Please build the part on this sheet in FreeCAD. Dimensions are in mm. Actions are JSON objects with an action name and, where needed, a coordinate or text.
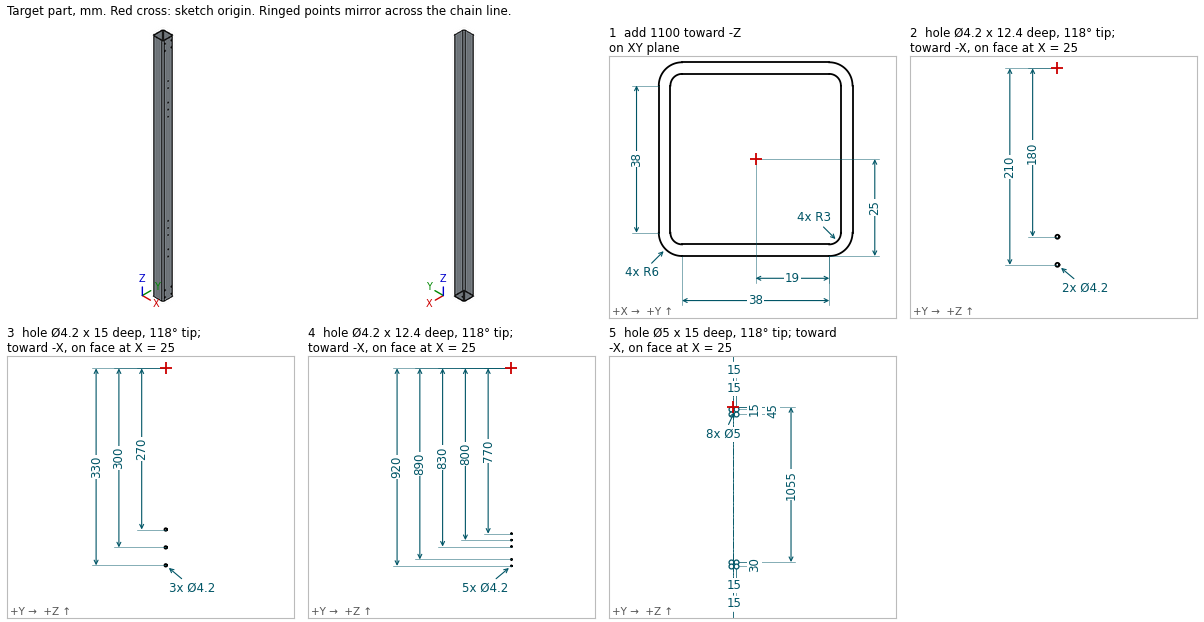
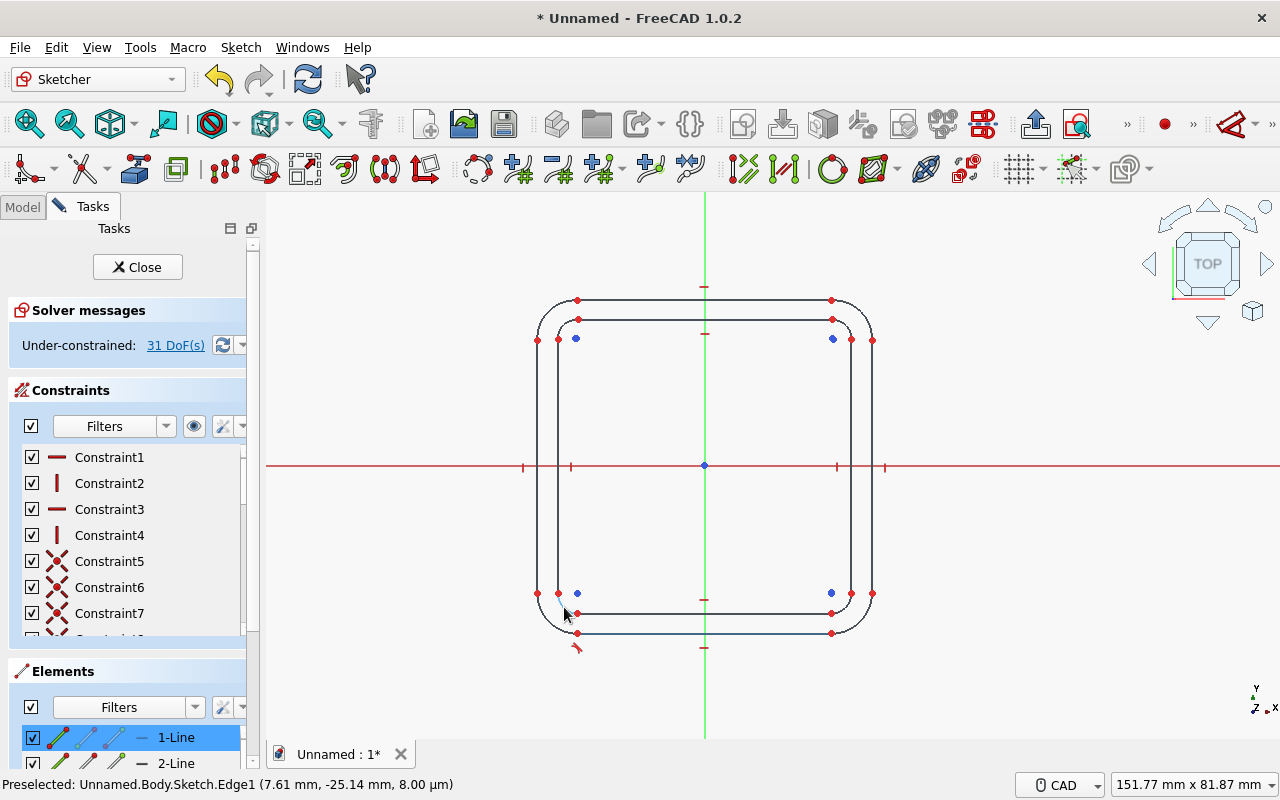
{"action": "left_click", "coordinate": [850, 629]}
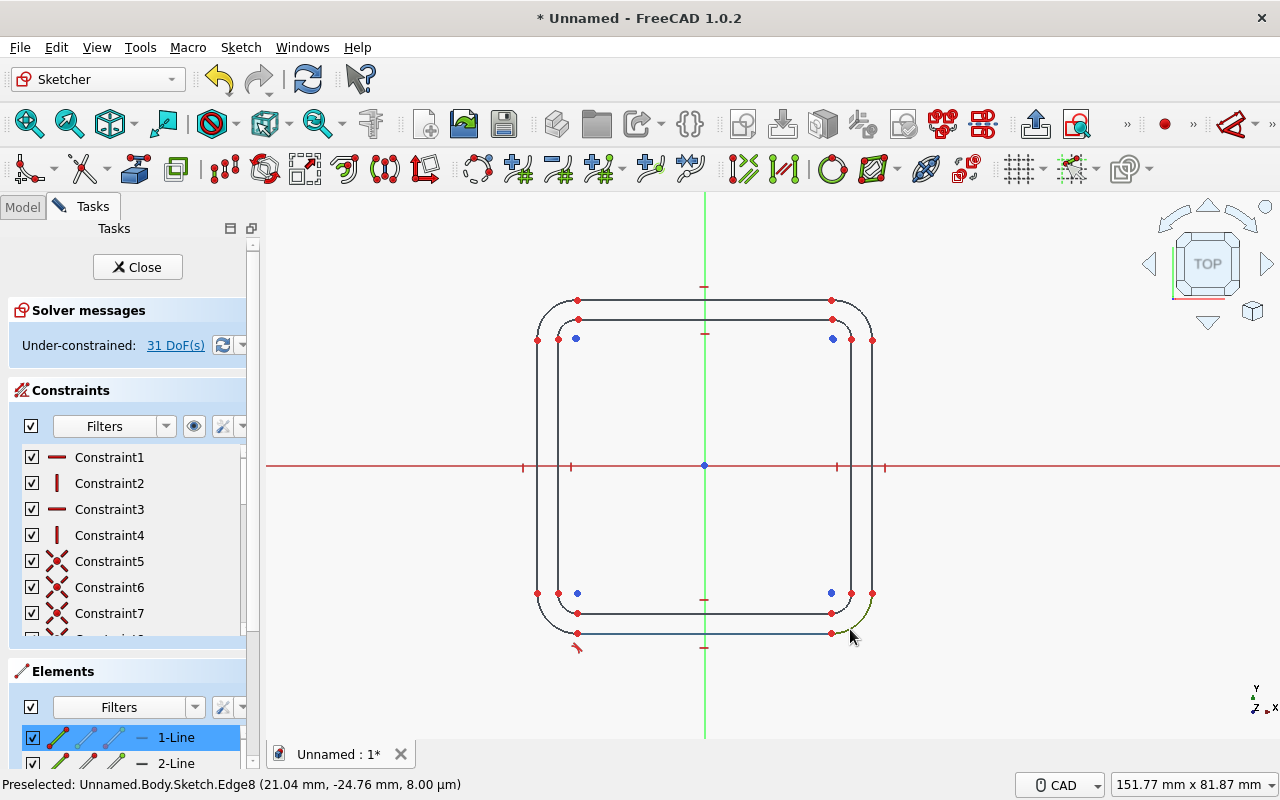
{"action": "key", "text": "t"}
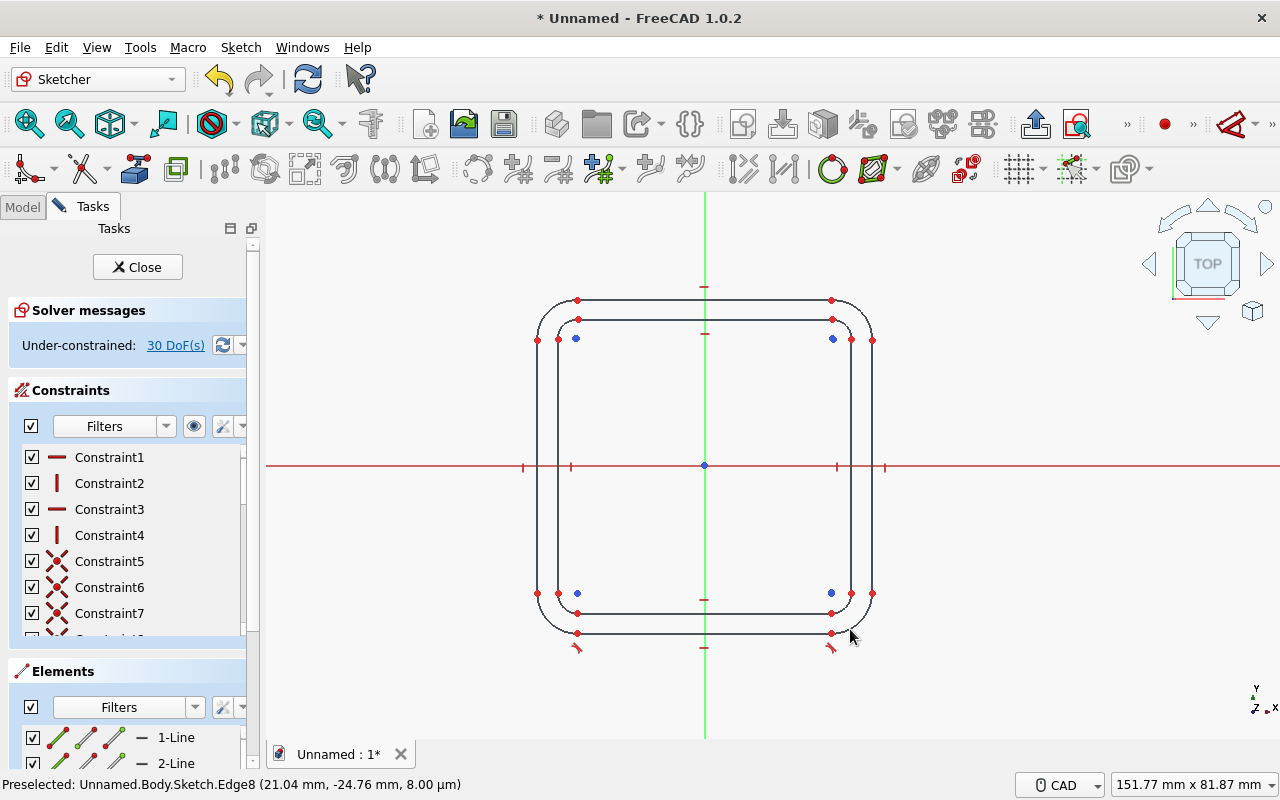
{"action": "left_click", "coordinate": [537, 518]}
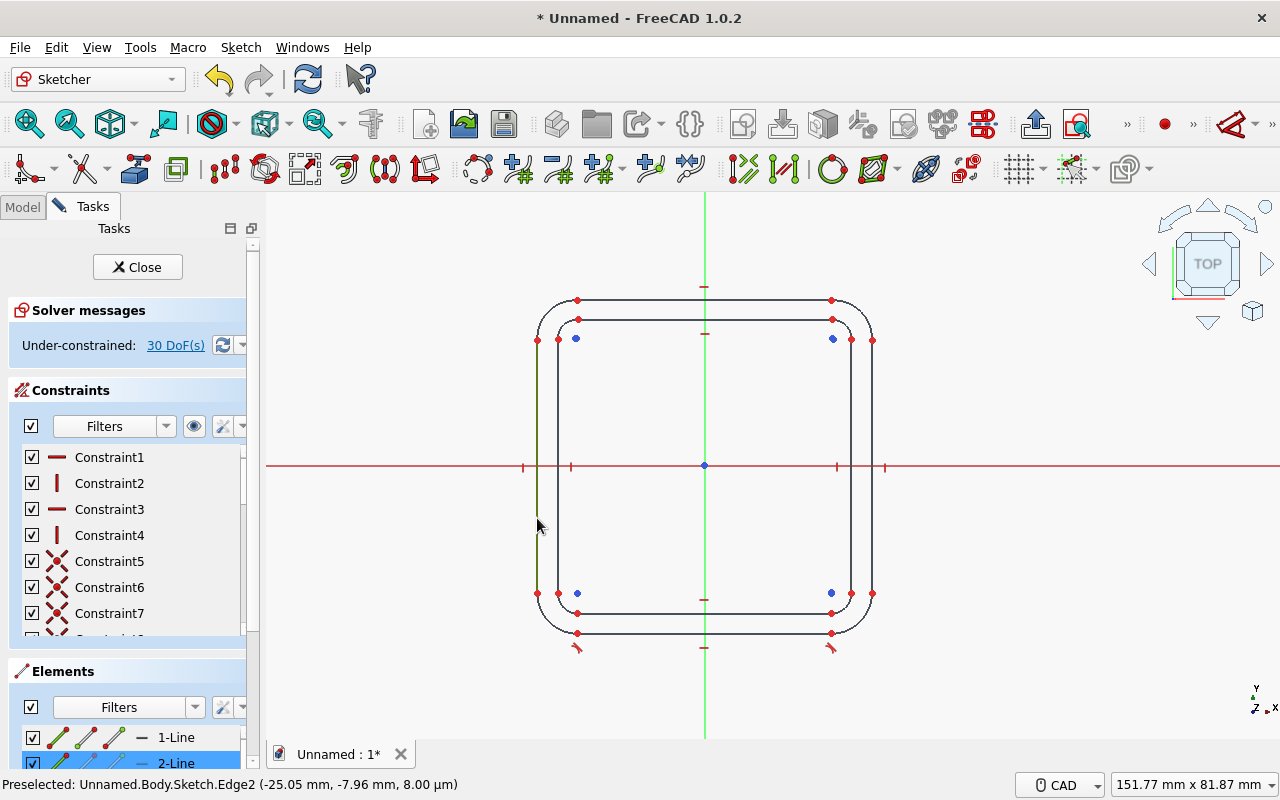
{"action": "left_click", "coordinate": [542, 612]}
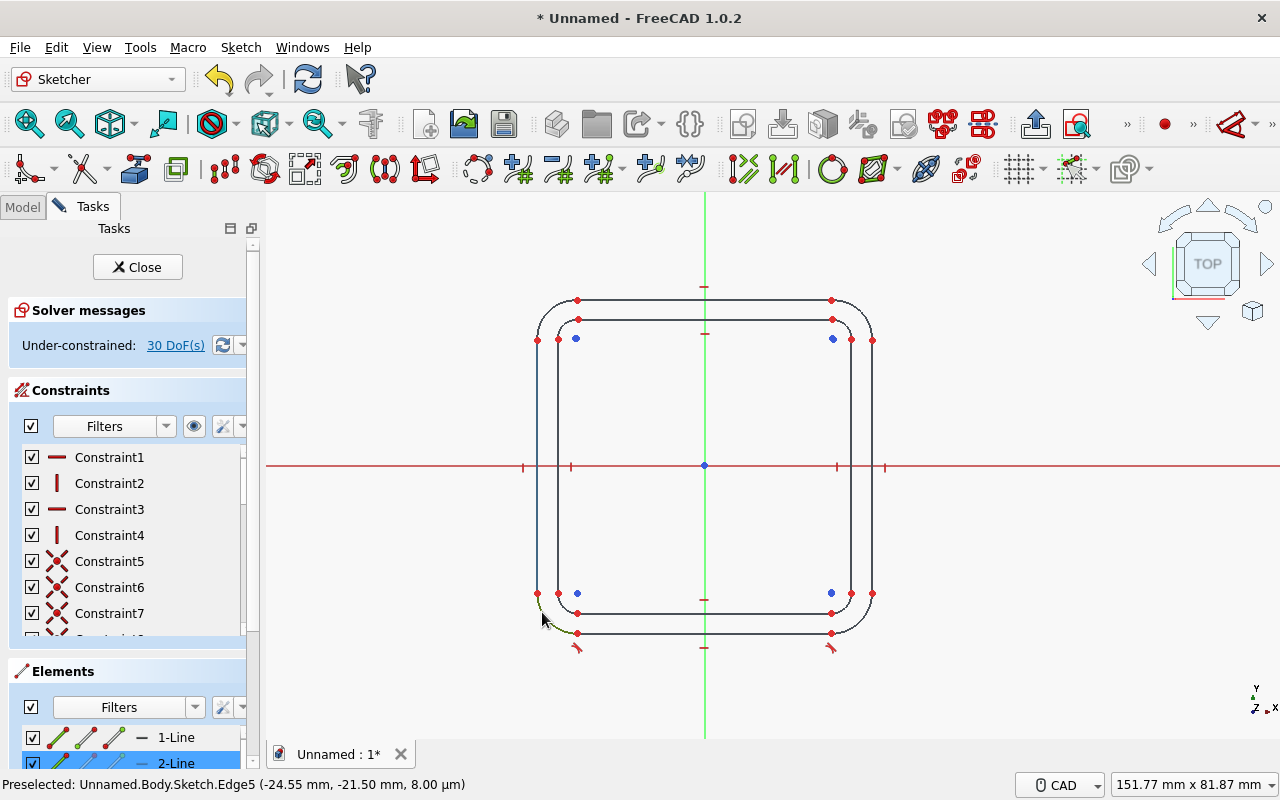
{"action": "key", "text": "t"}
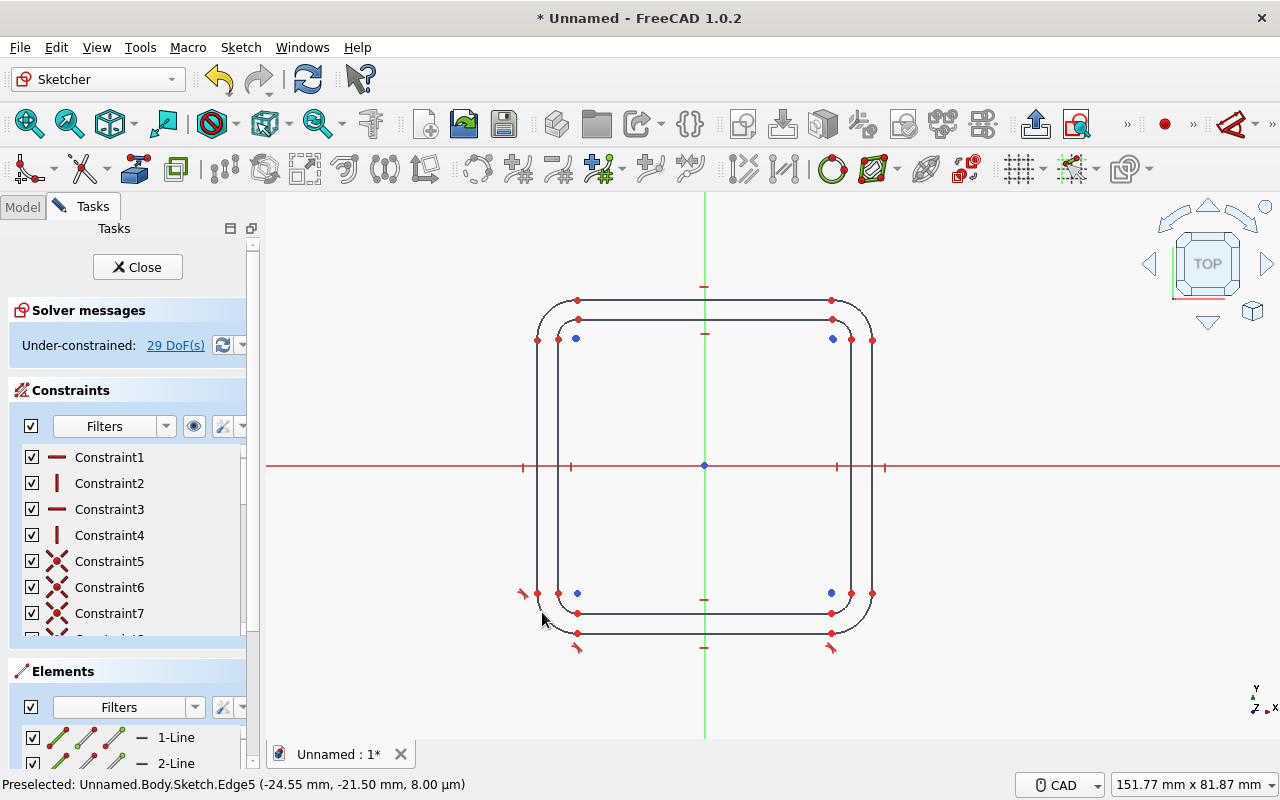
{"action": "left_click", "coordinate": [537, 518]}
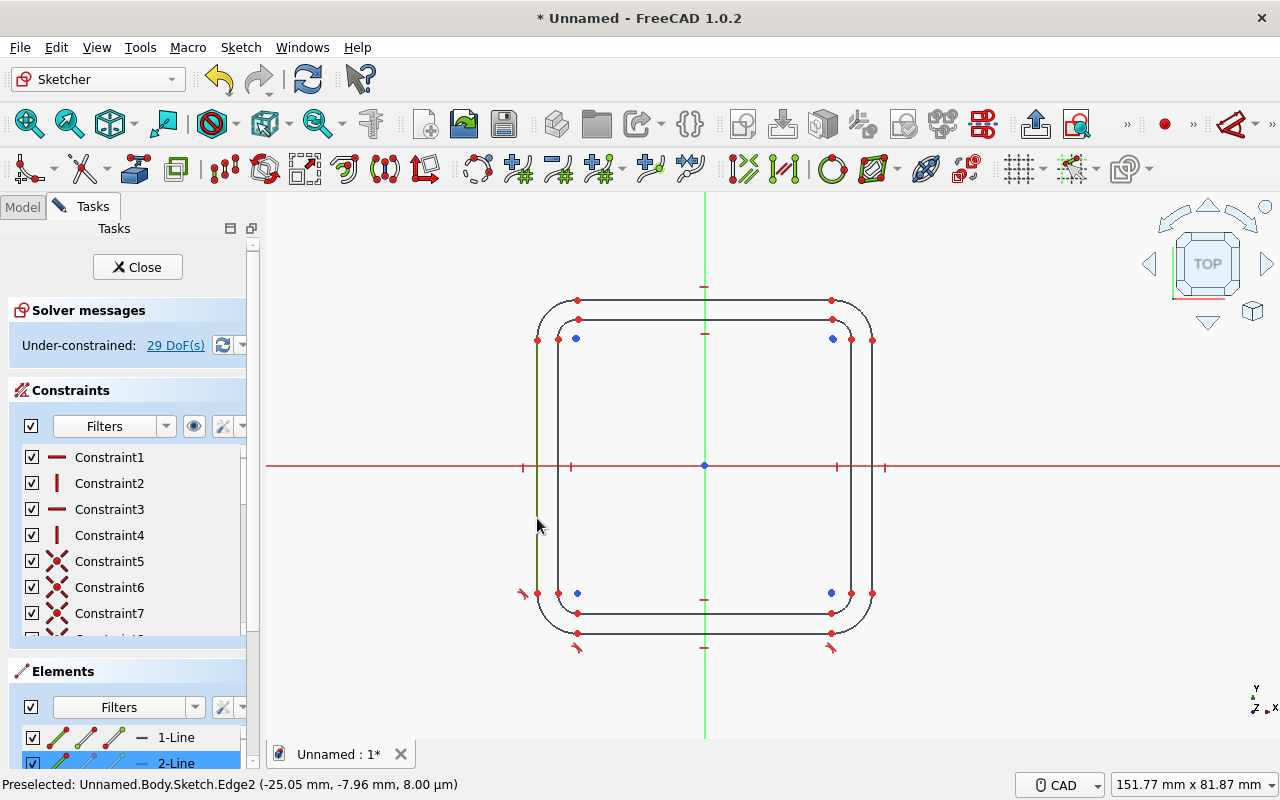
{"action": "left_click", "coordinate": [559, 304]}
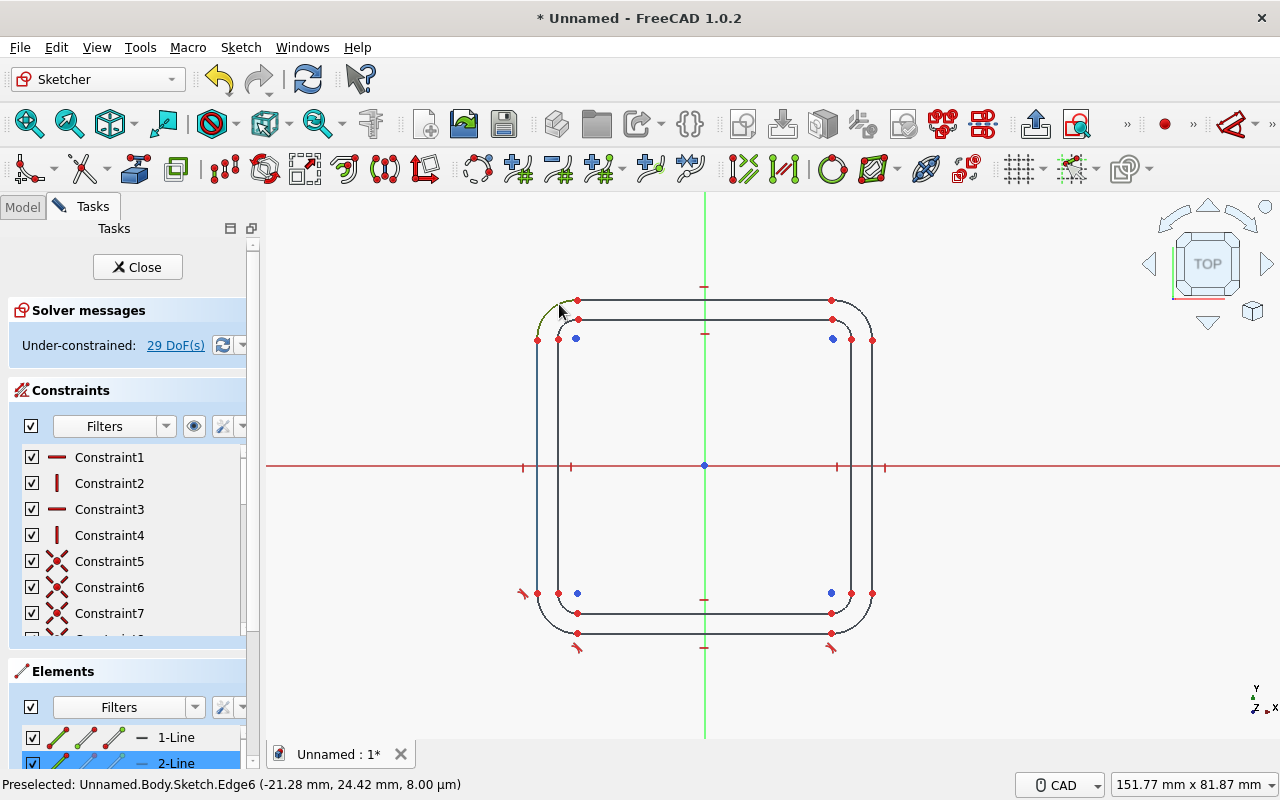
{"action": "key", "text": "t"}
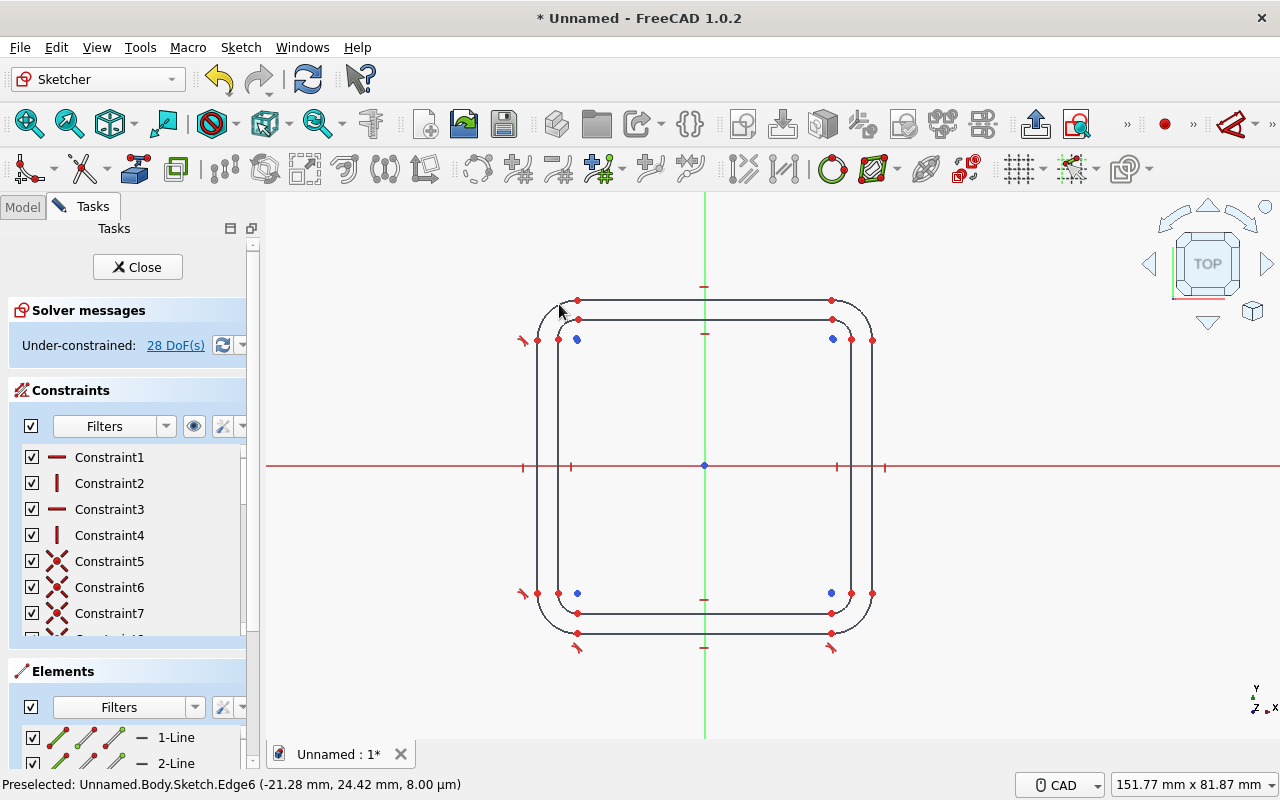
{"action": "left_click", "coordinate": [654, 300]}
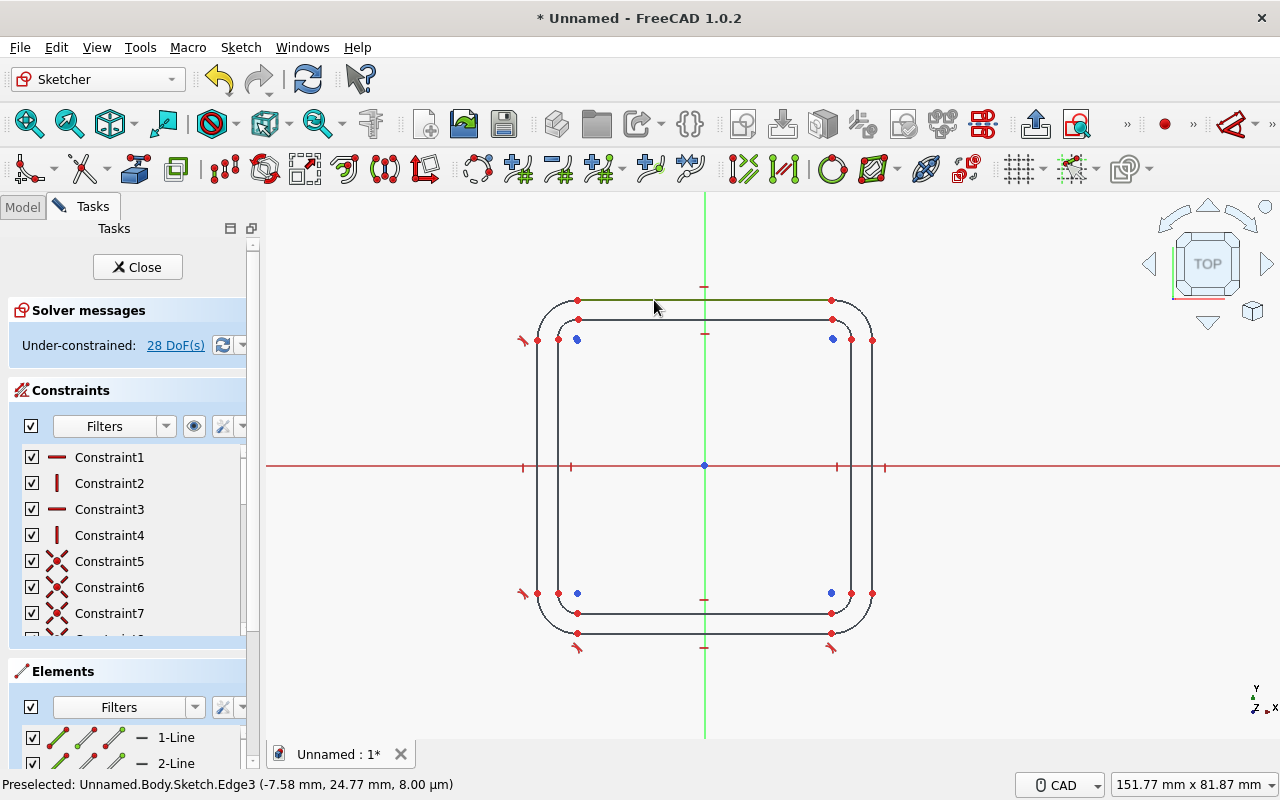
{"action": "left_click", "coordinate": [559, 305]}